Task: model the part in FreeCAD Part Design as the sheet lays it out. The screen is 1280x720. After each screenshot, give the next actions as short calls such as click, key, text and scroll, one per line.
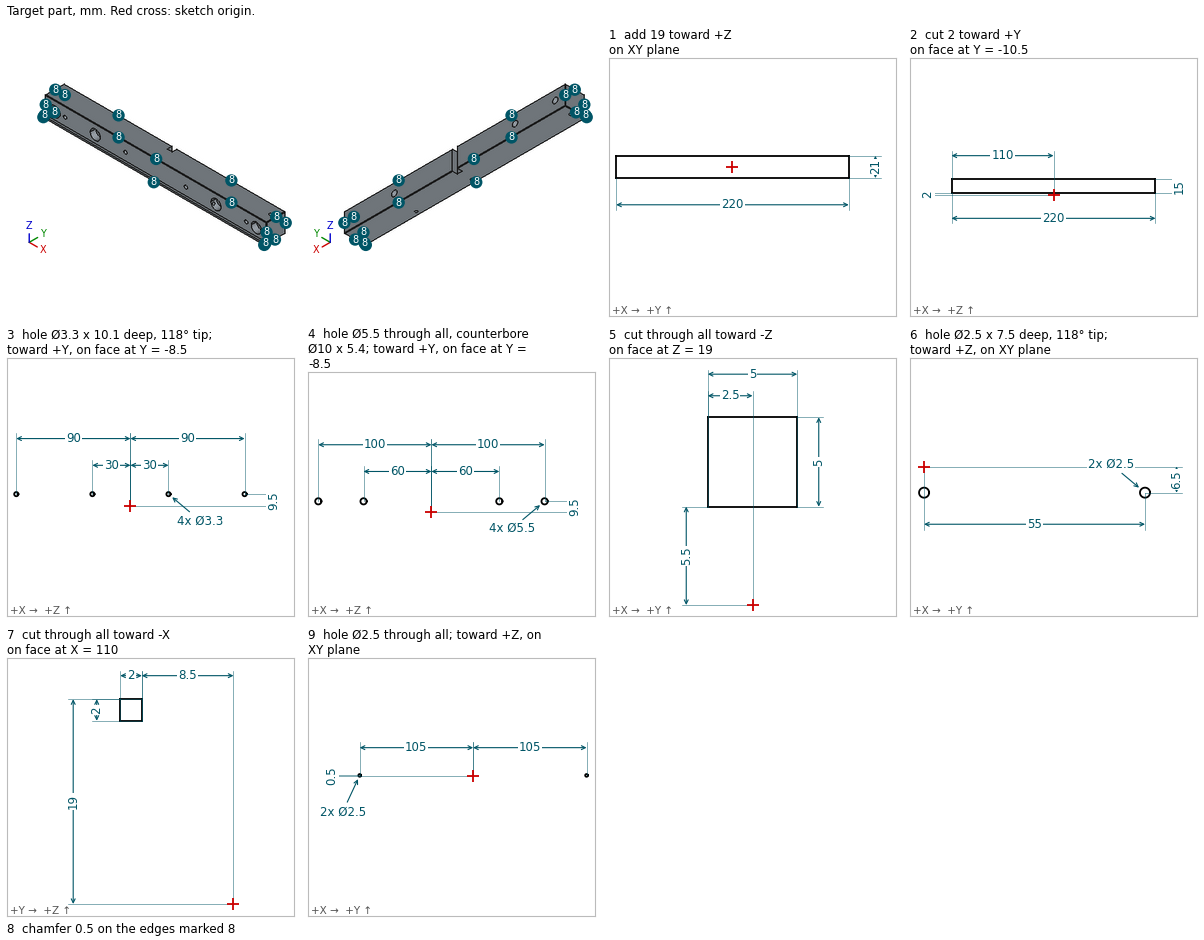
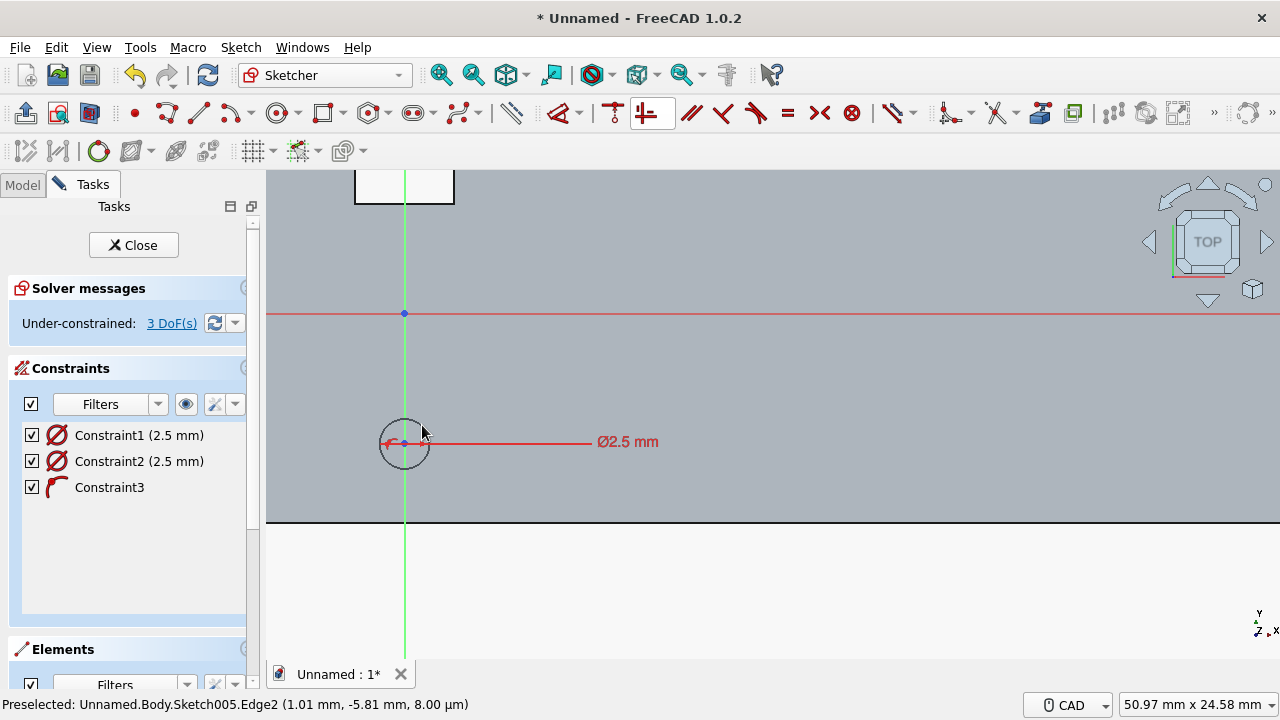
scroll(404, 443, down, 3)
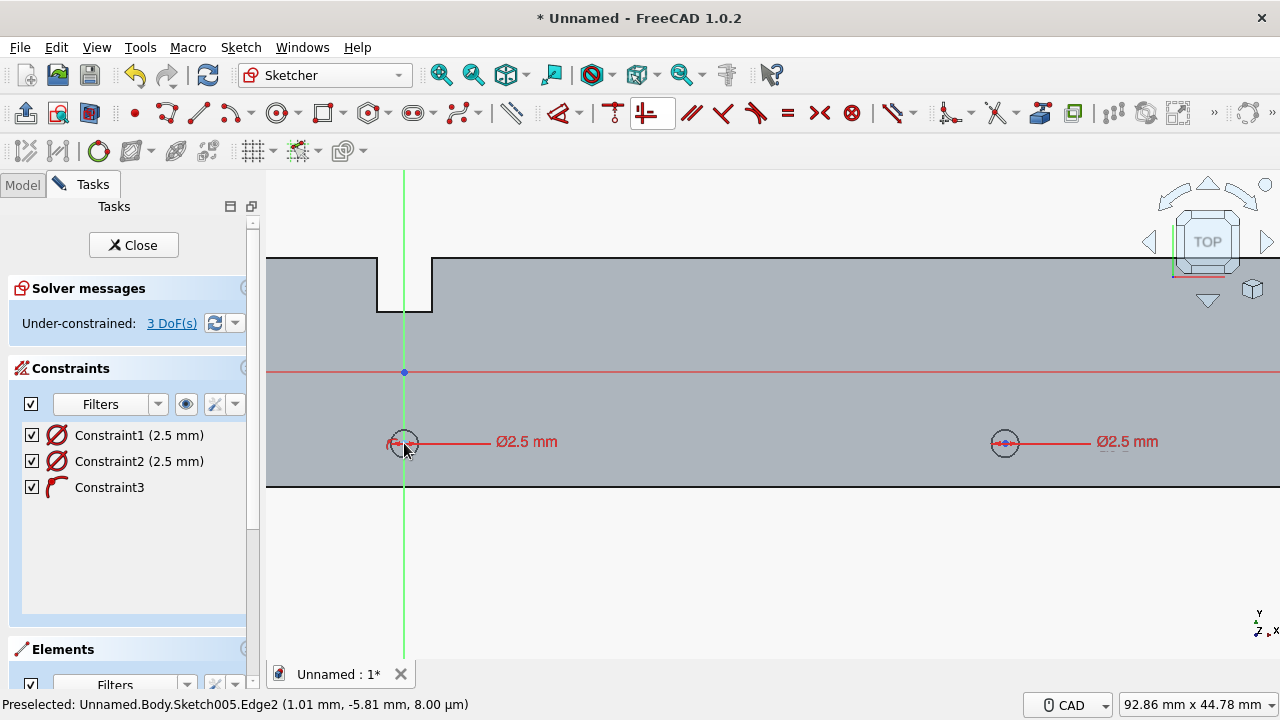
click(1005, 444)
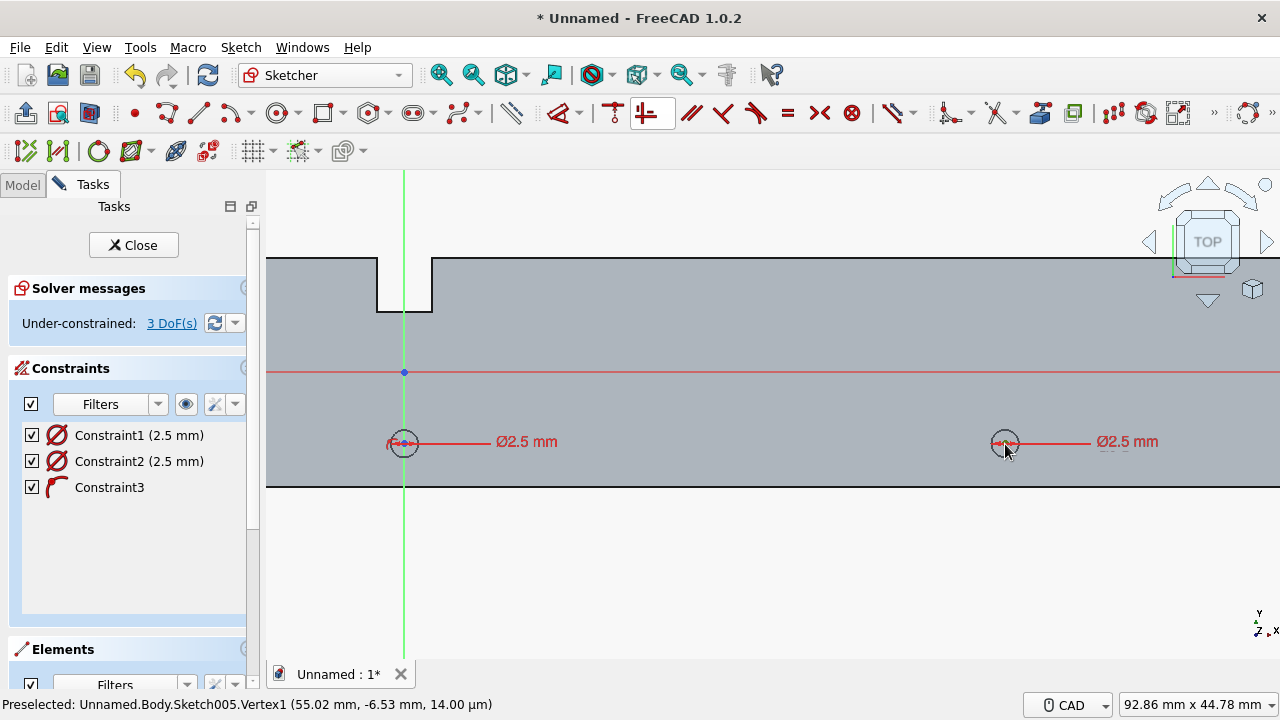
click(404, 444)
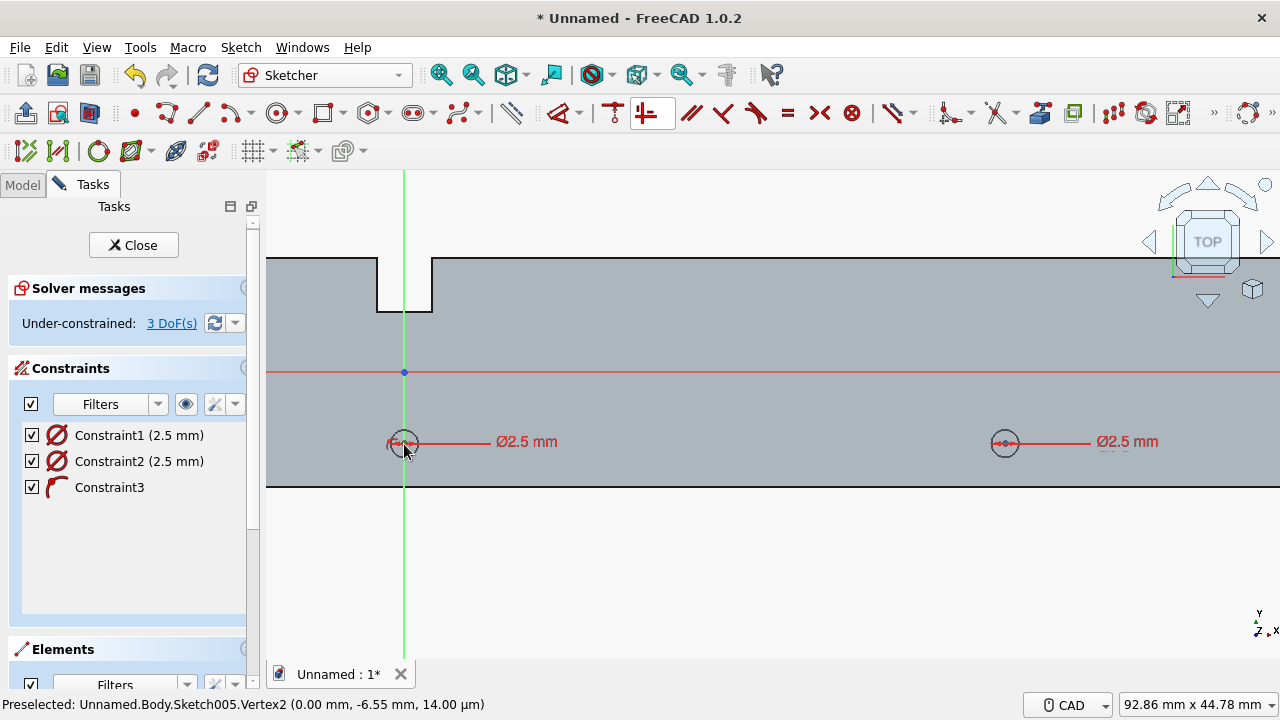
key(h)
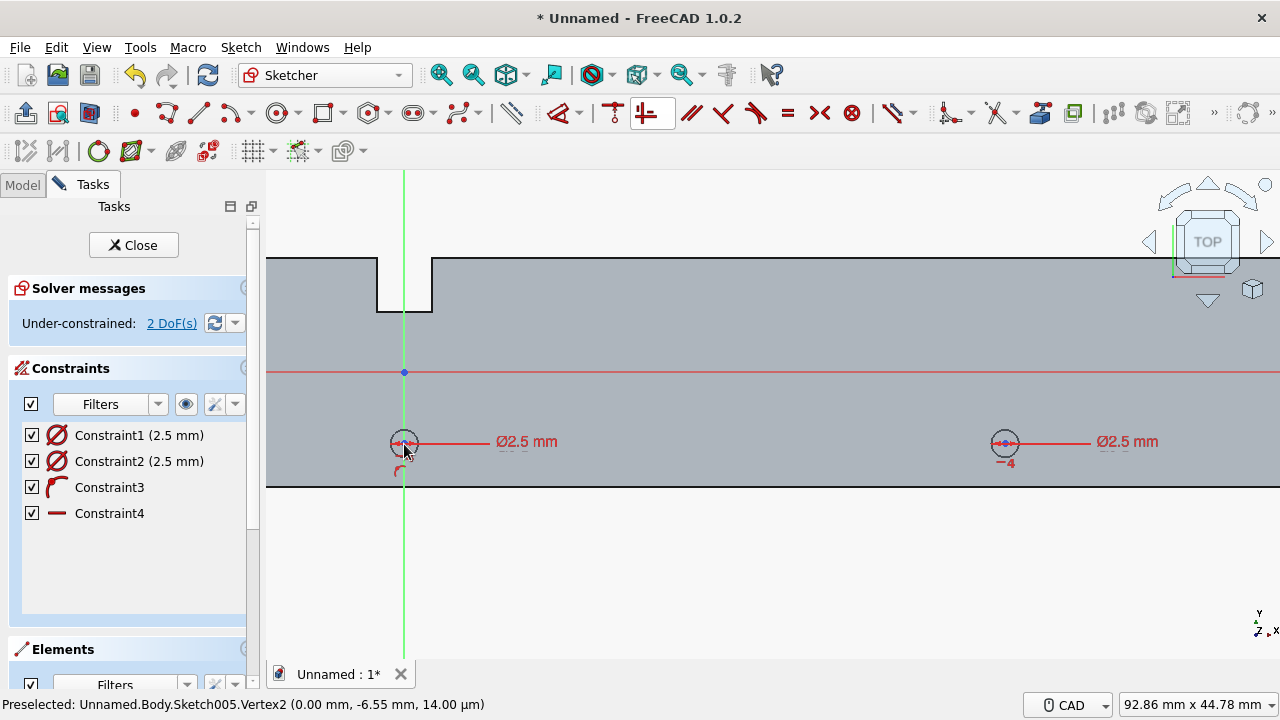
click(558, 114)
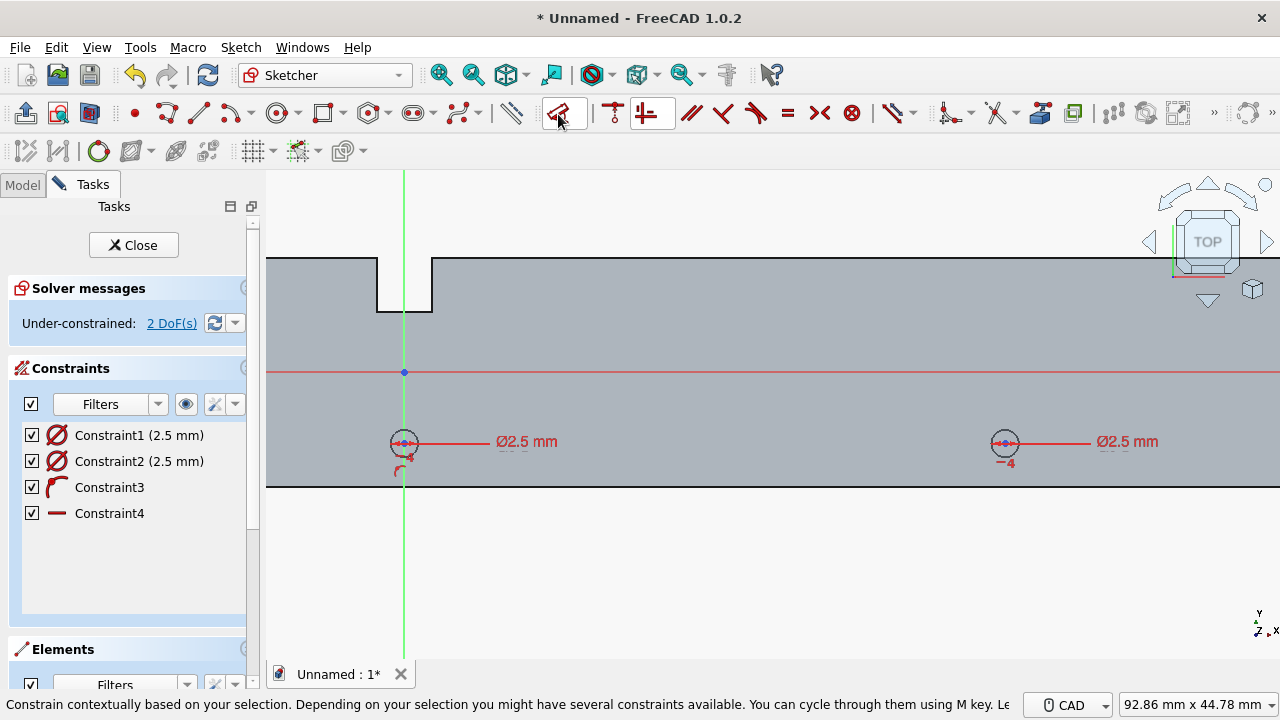
click(1005, 444)
click(705, 338)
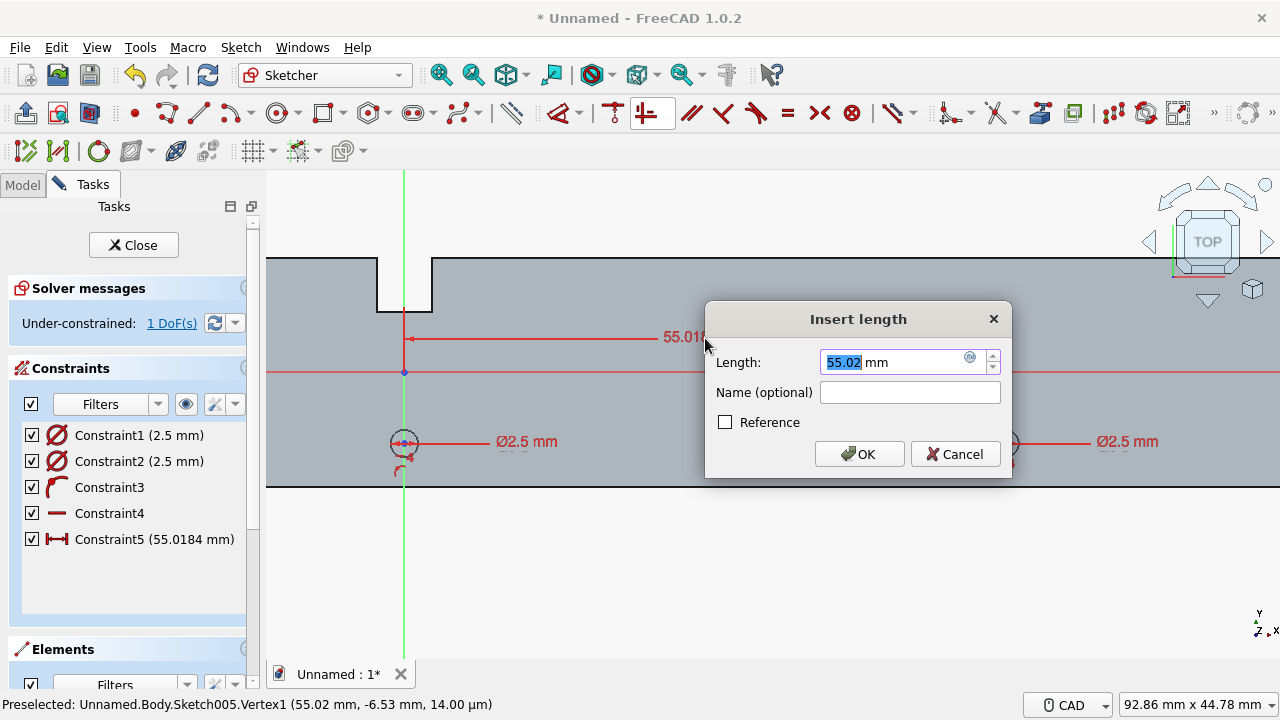
text(55)
key(Return)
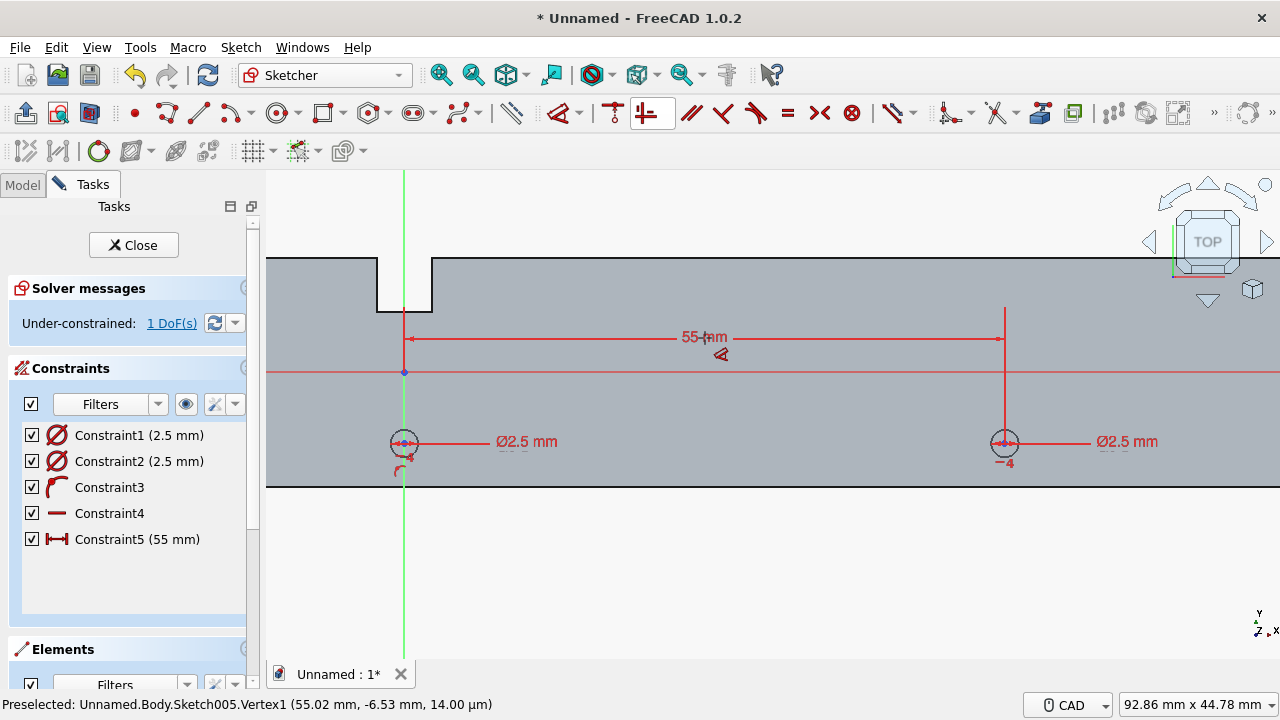
click(1005, 444)
click(1039, 408)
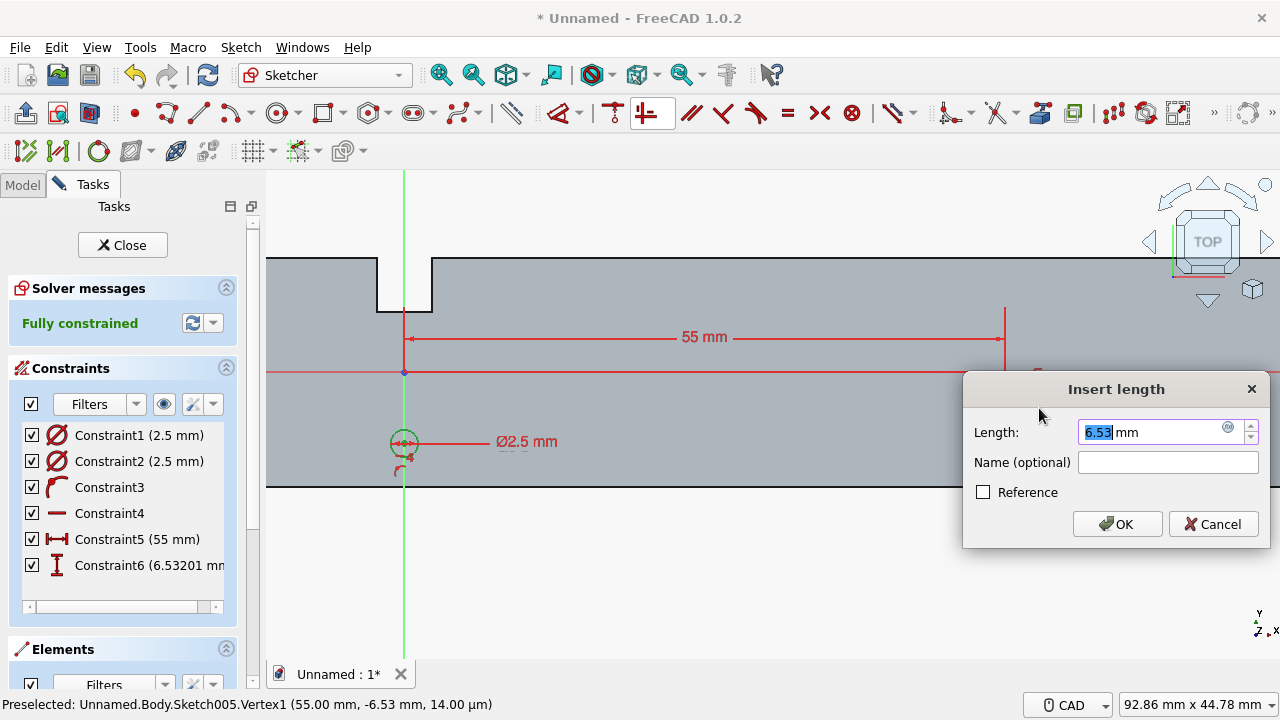
text(6.5)
key(Return)
key(Escape)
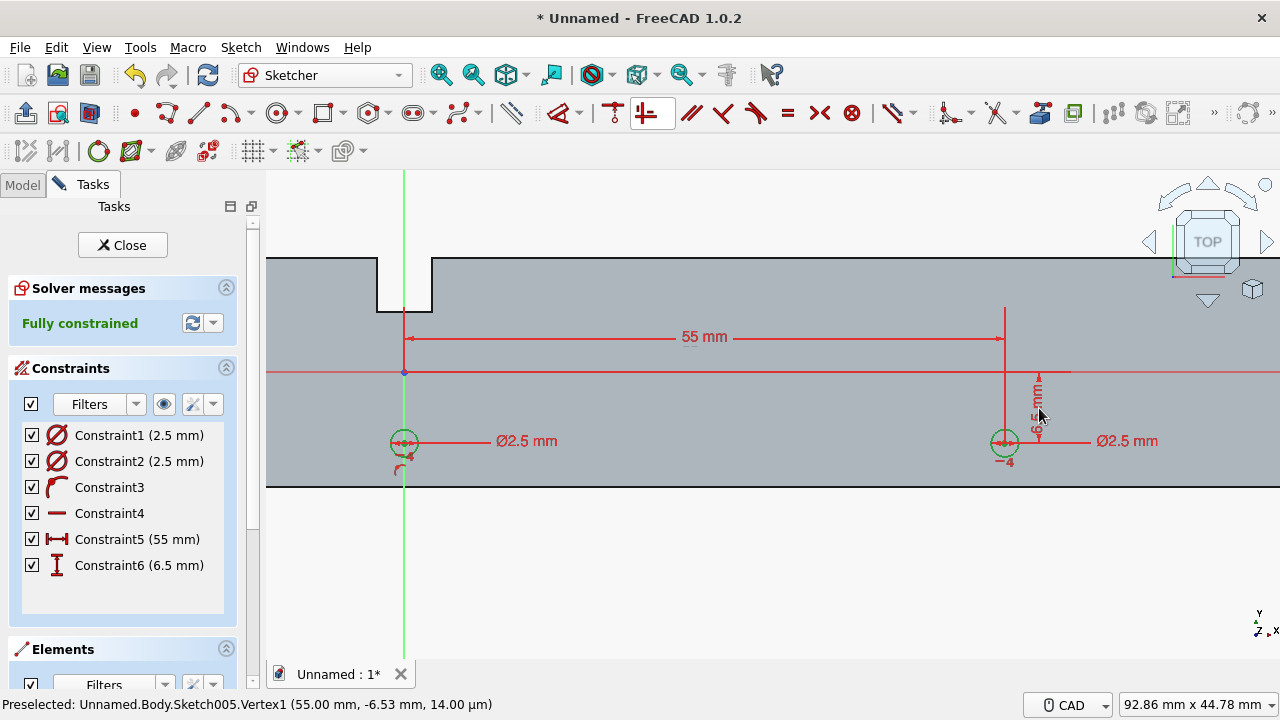
click(123, 245)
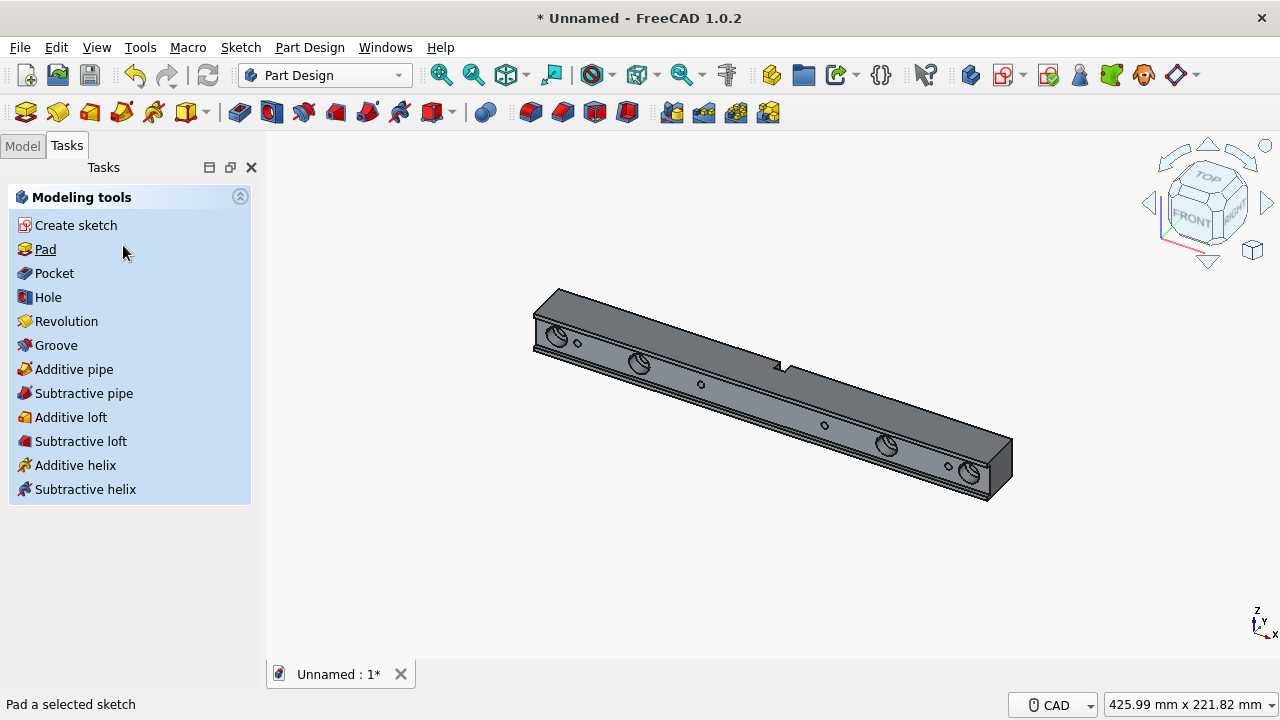
click(272, 112)